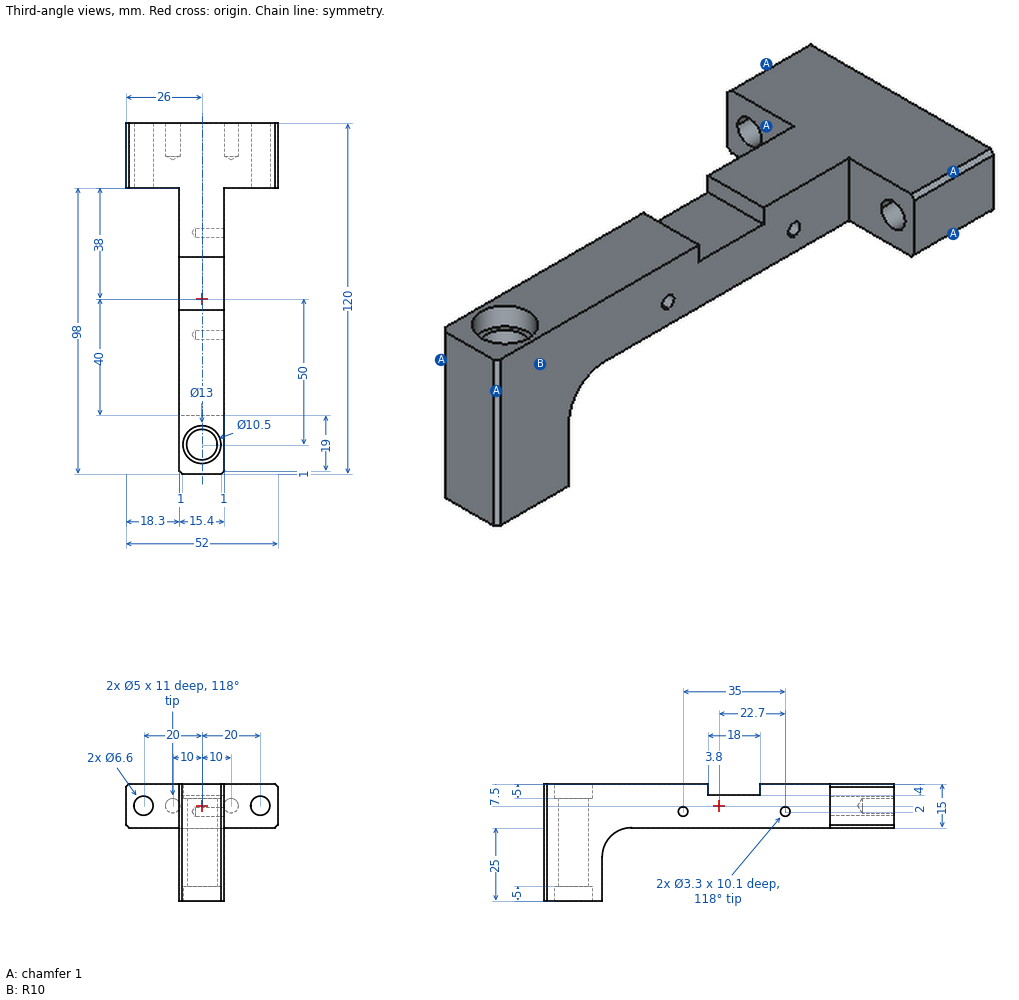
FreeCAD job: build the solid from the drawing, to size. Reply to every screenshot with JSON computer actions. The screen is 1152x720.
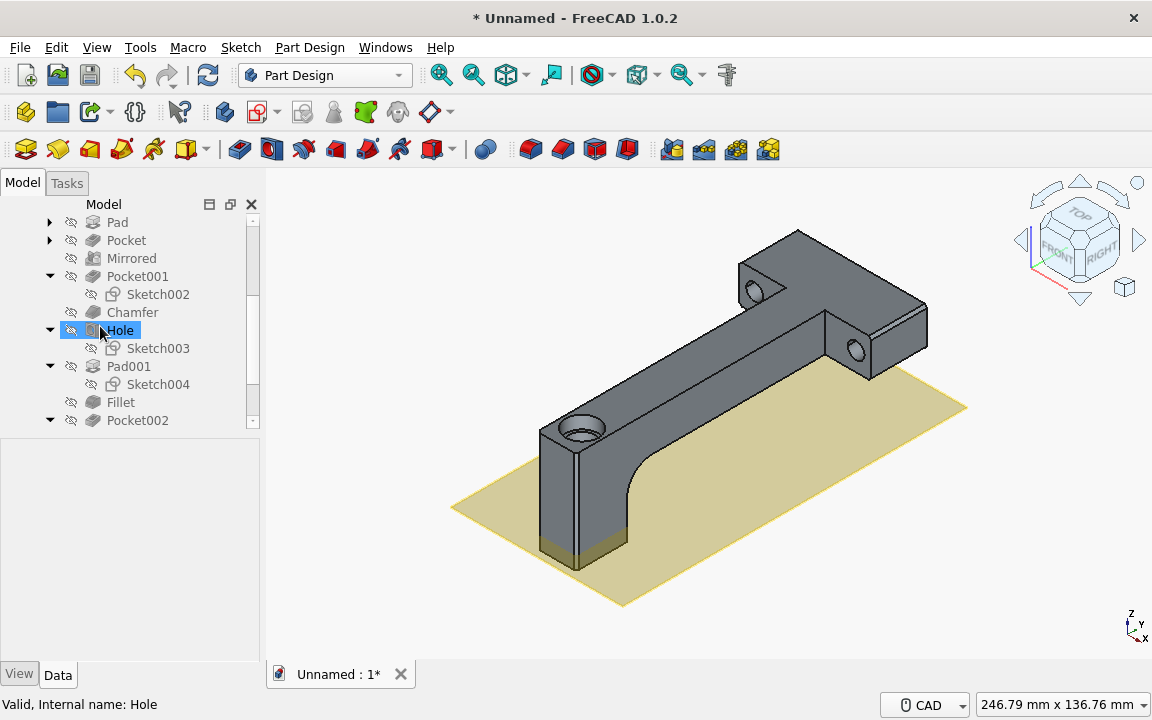
{"action": "scroll", "coordinate": [140, 326], "scroll_direction": "up", "scroll_amount": 15}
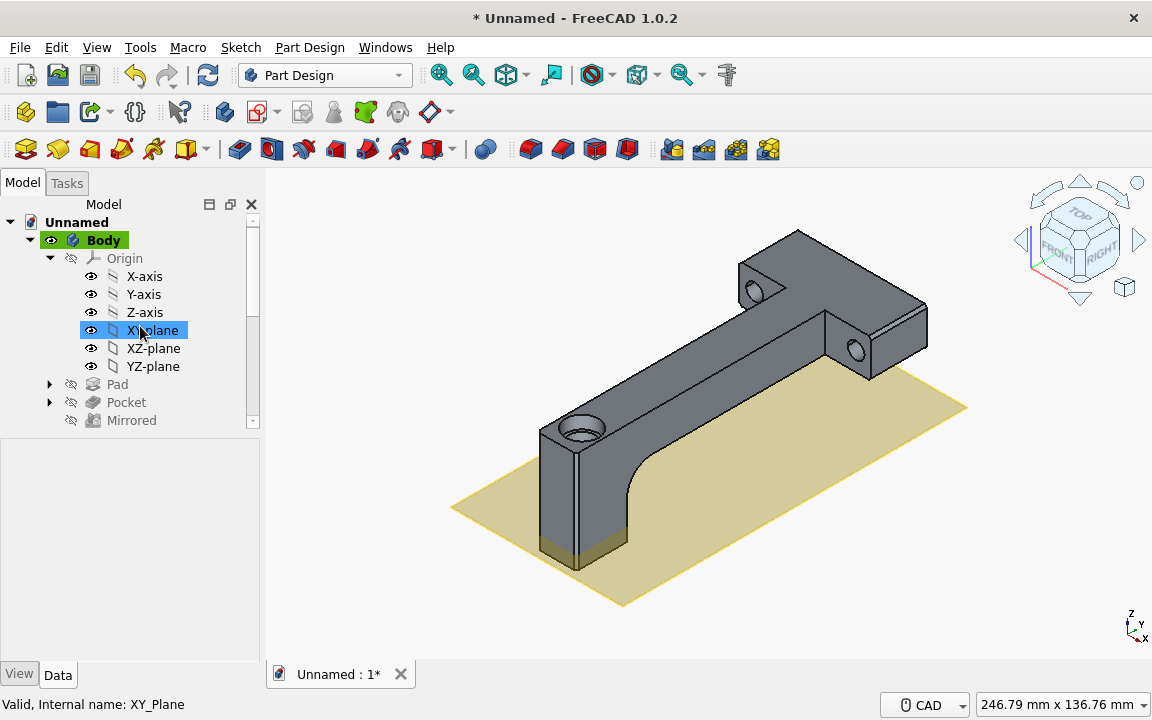
{"action": "scroll", "coordinate": [100, 326], "scroll_direction": "down", "scroll_amount": 6}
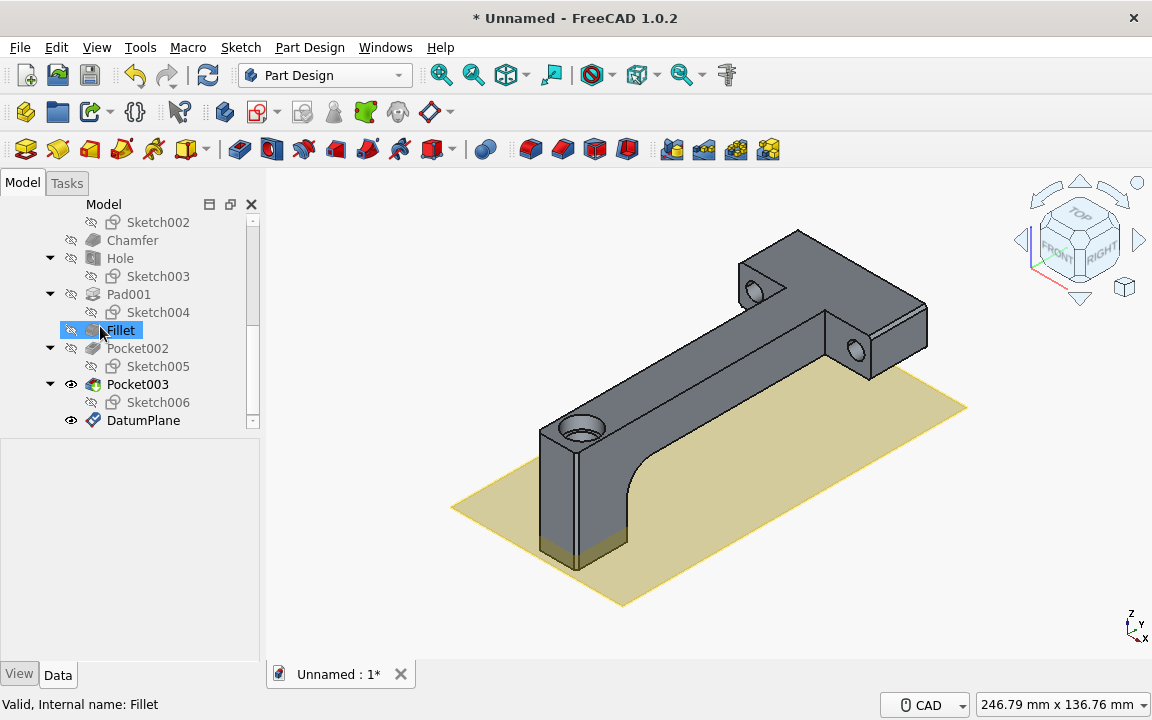
{"action": "left_click", "coordinate": [116, 420]}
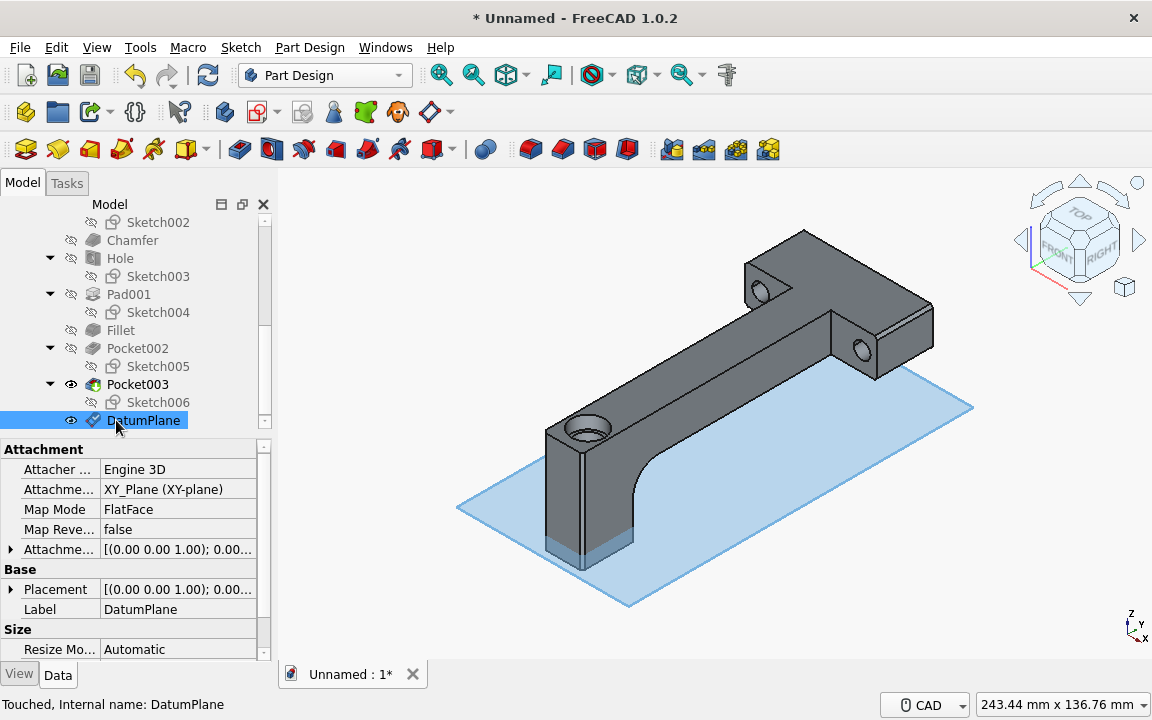
{"action": "left_click", "coordinate": [258, 112]}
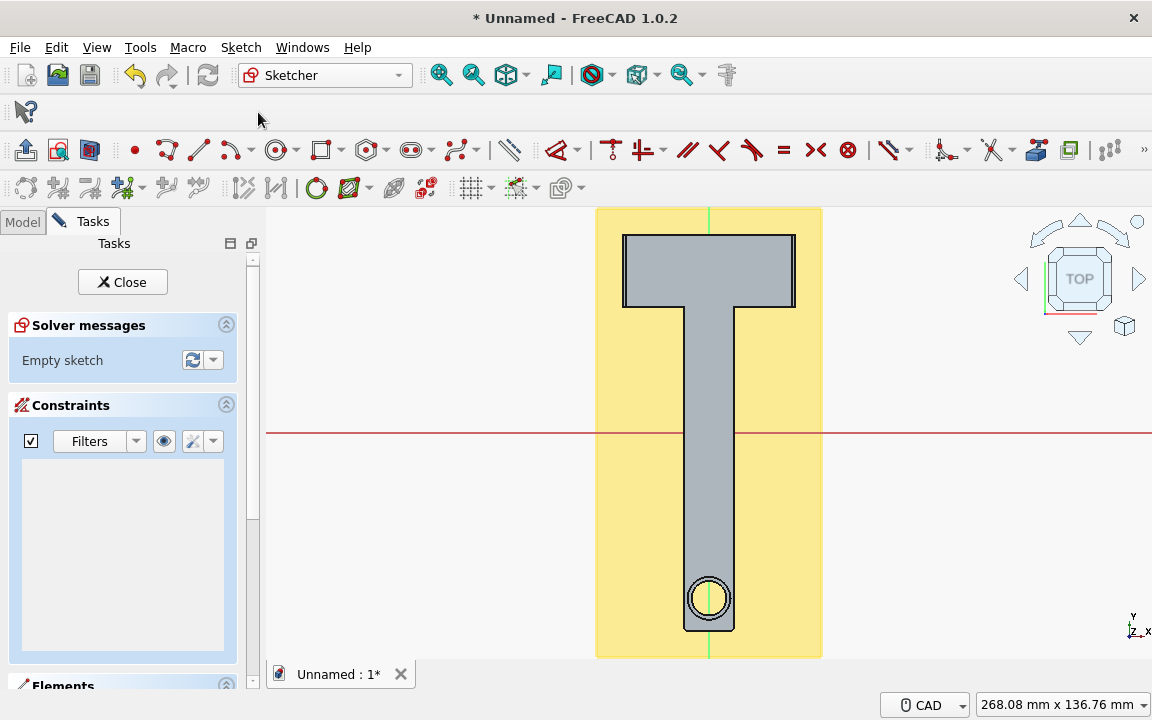
{"action": "left_click", "coordinate": [90, 150]}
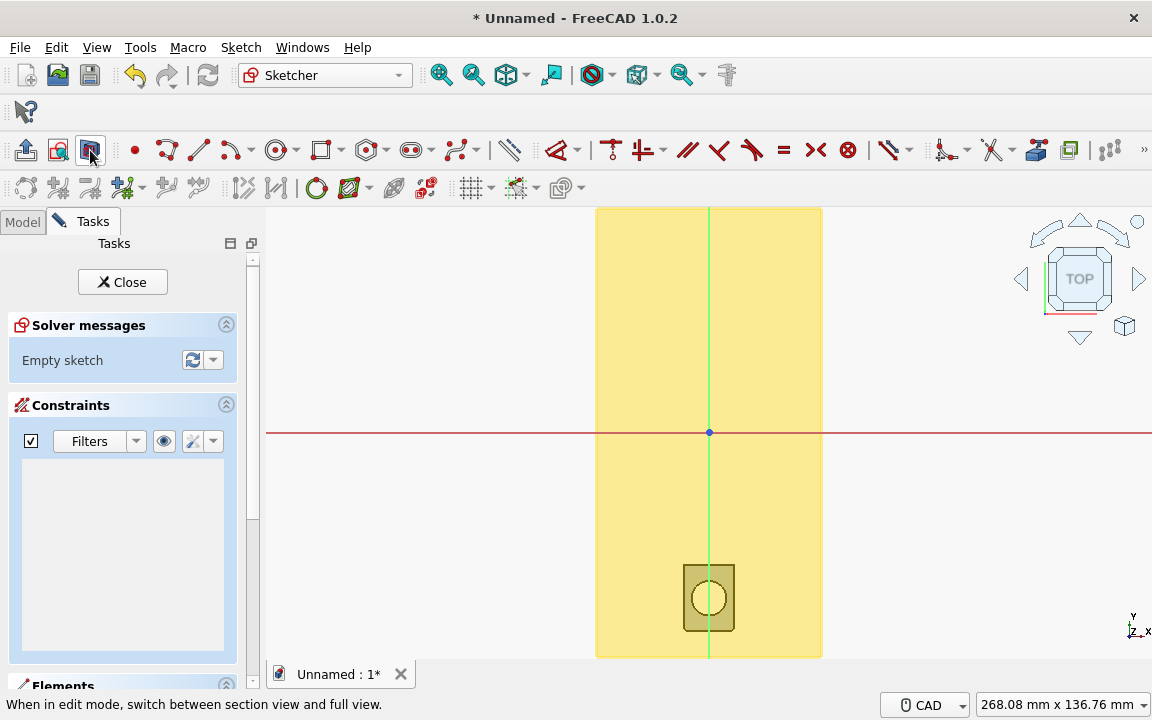
{"action": "scroll", "coordinate": [723, 631], "scroll_direction": "up", "scroll_amount": 9}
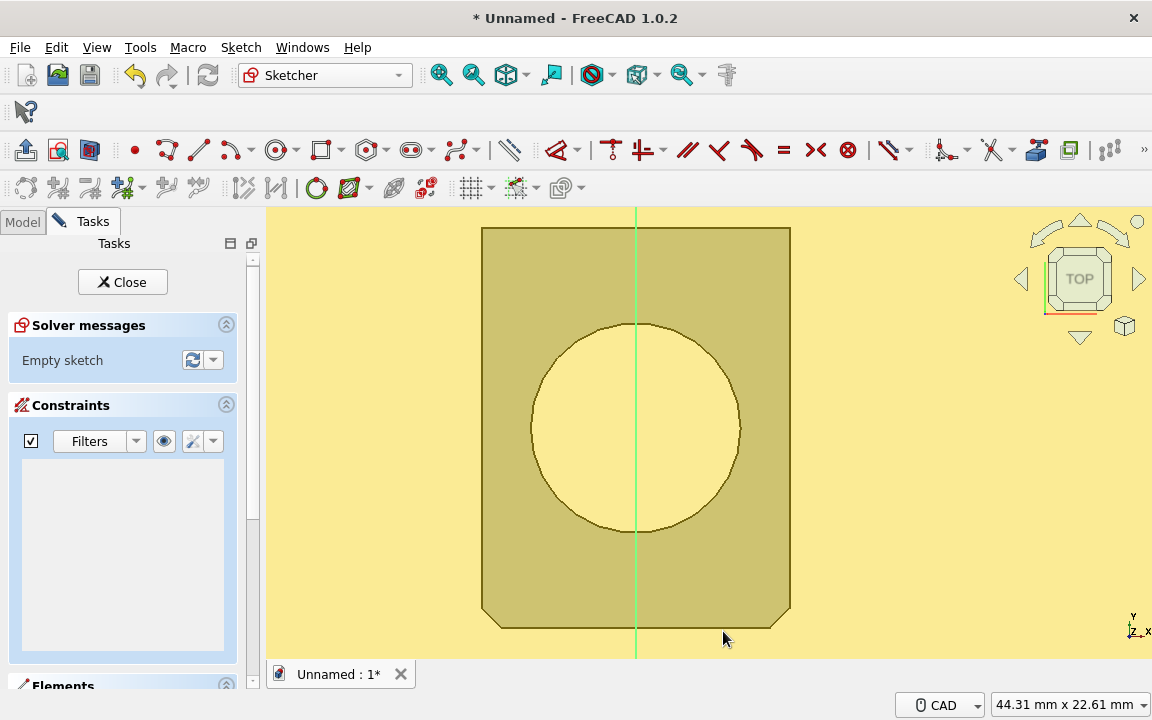
{"action": "left_click", "coordinate": [276, 150]}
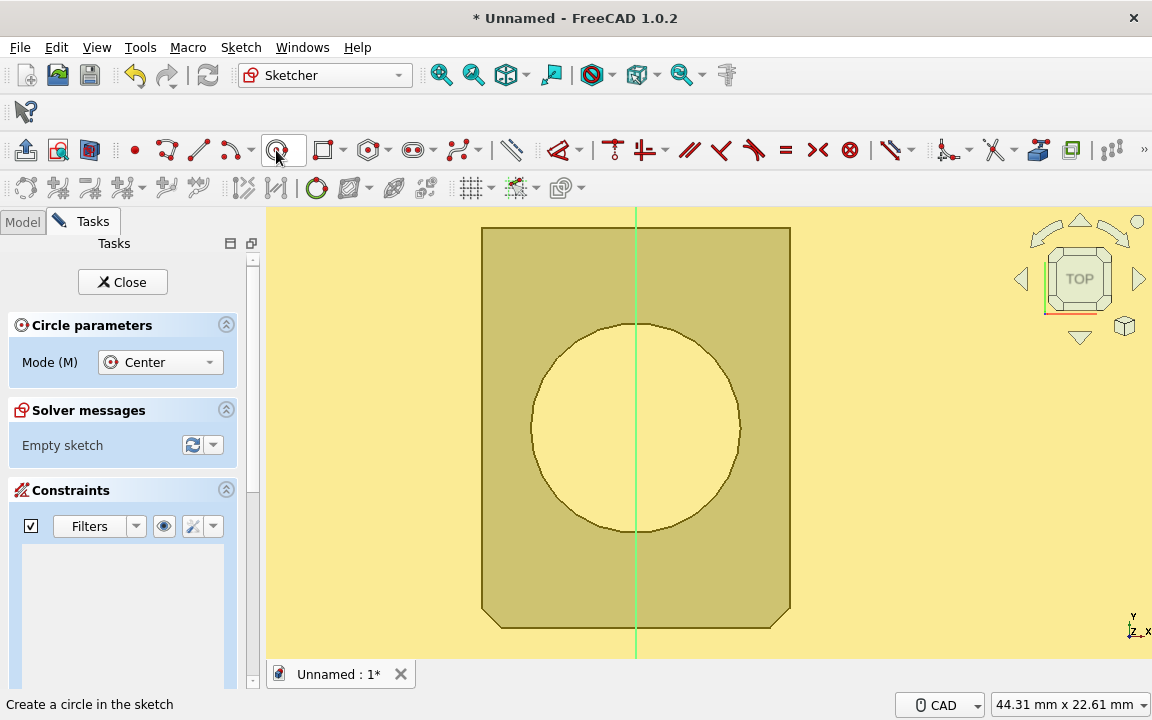
{"action": "left_click", "coordinate": [636, 428]}
{"action": "mouse_move", "coordinate": [728, 336]}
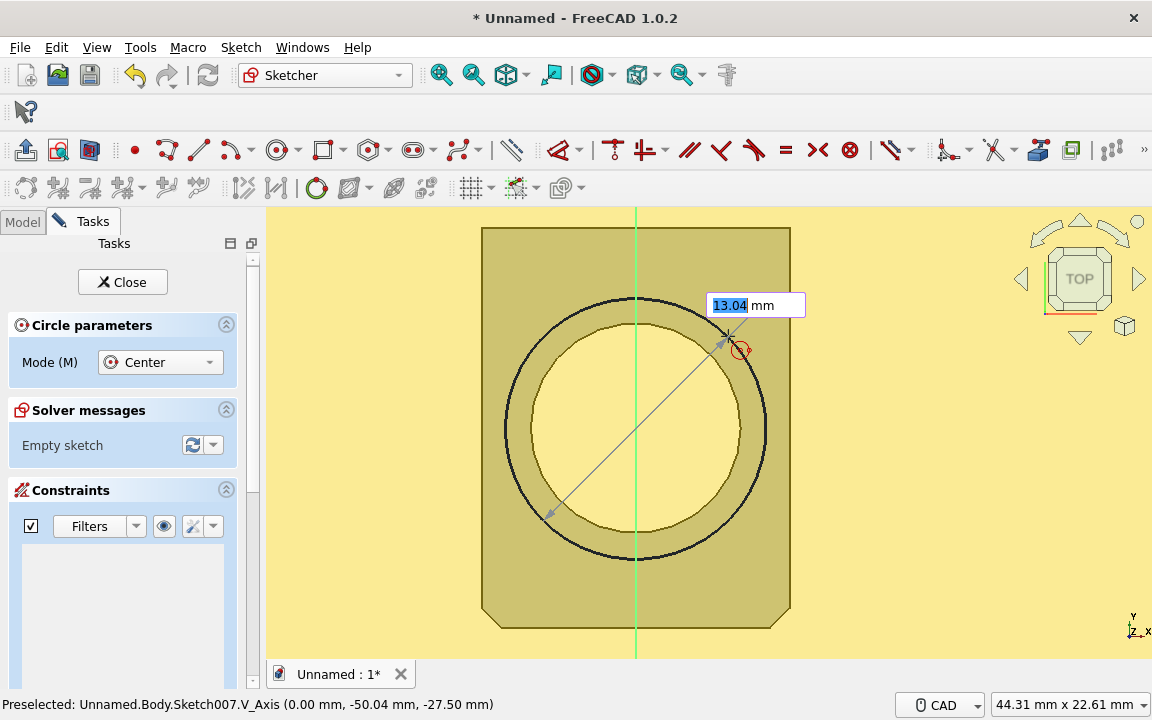
{"action": "type", "text": "13"}
{"action": "key", "text": "Return"}
{"action": "key", "text": "Escape"}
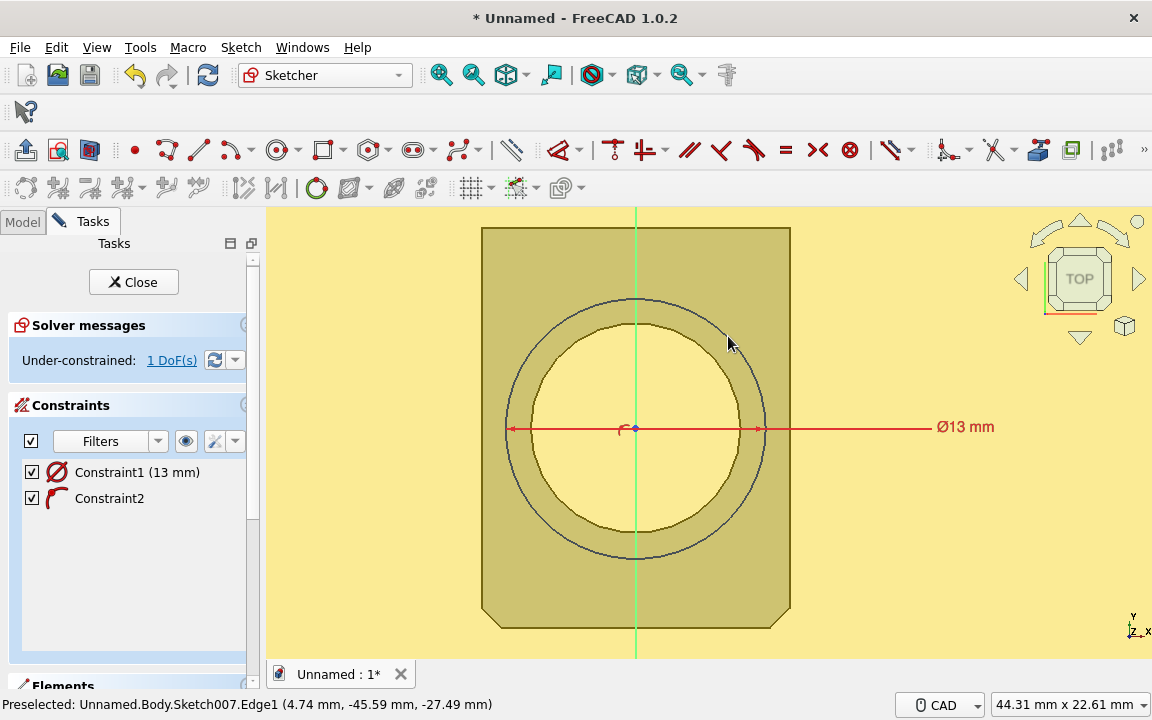
{"action": "left_click", "coordinate": [558, 150]}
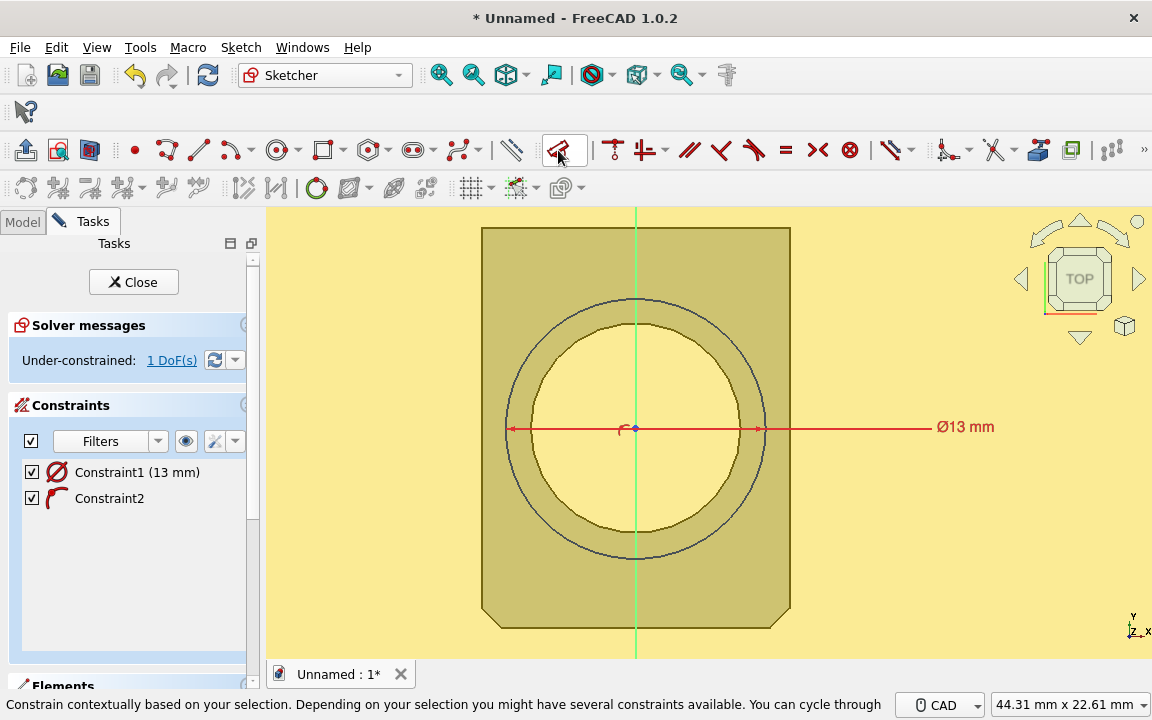
{"action": "left_click", "coordinate": [636, 429]}
{"action": "left_click", "coordinate": [670, 332]}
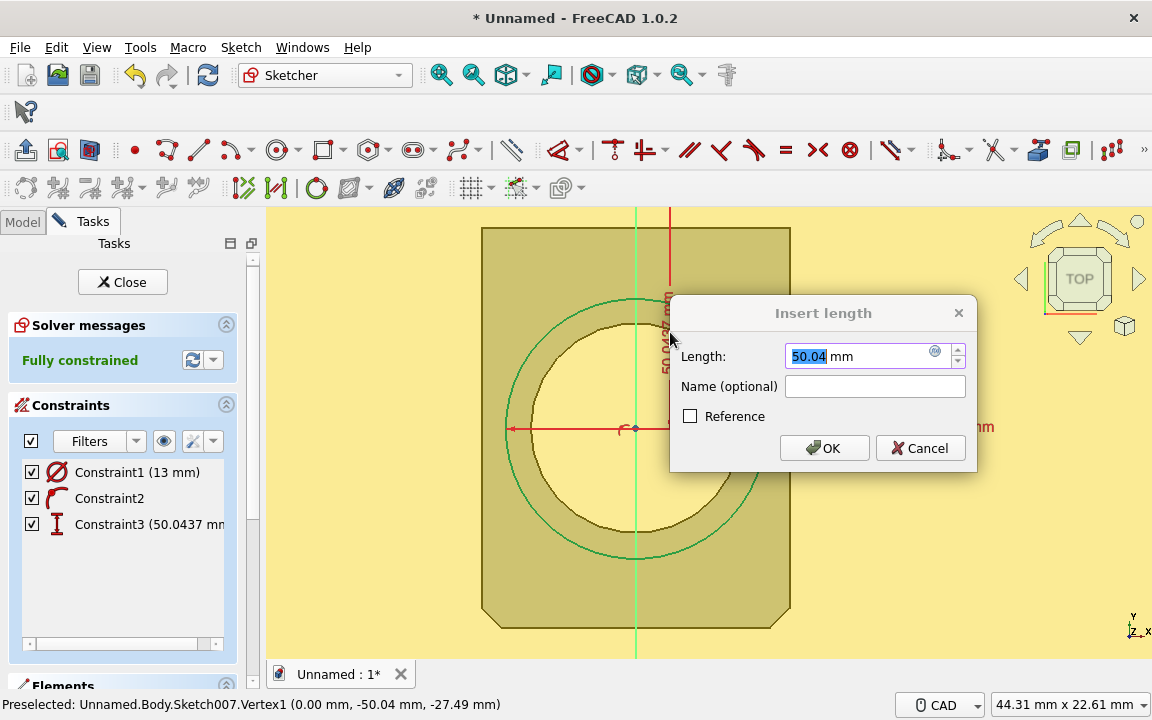
{"action": "type", "text": "50"}
{"action": "key", "text": "Return"}
{"action": "key", "text": "Escape"}